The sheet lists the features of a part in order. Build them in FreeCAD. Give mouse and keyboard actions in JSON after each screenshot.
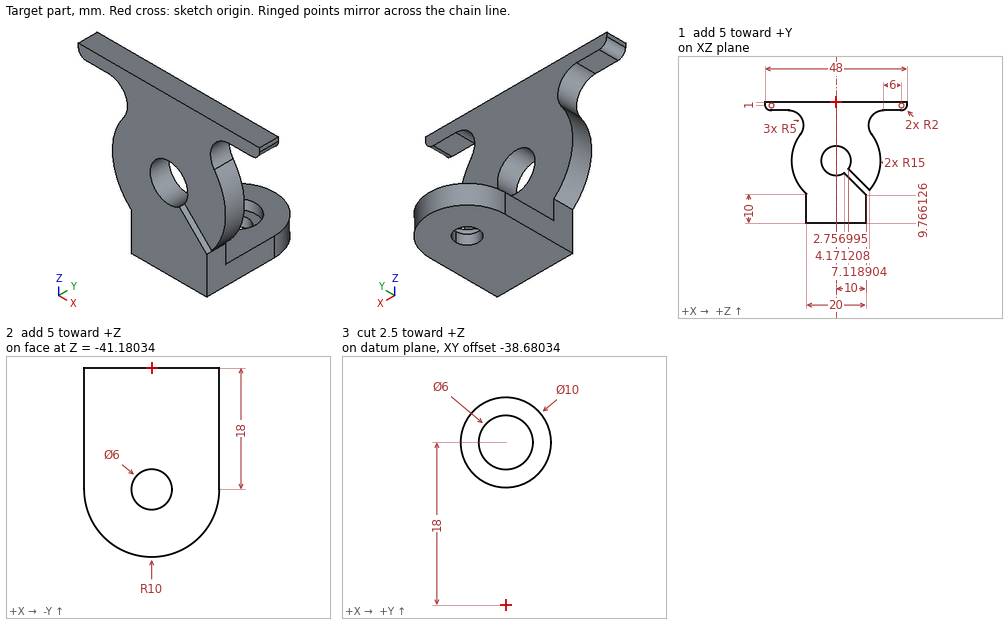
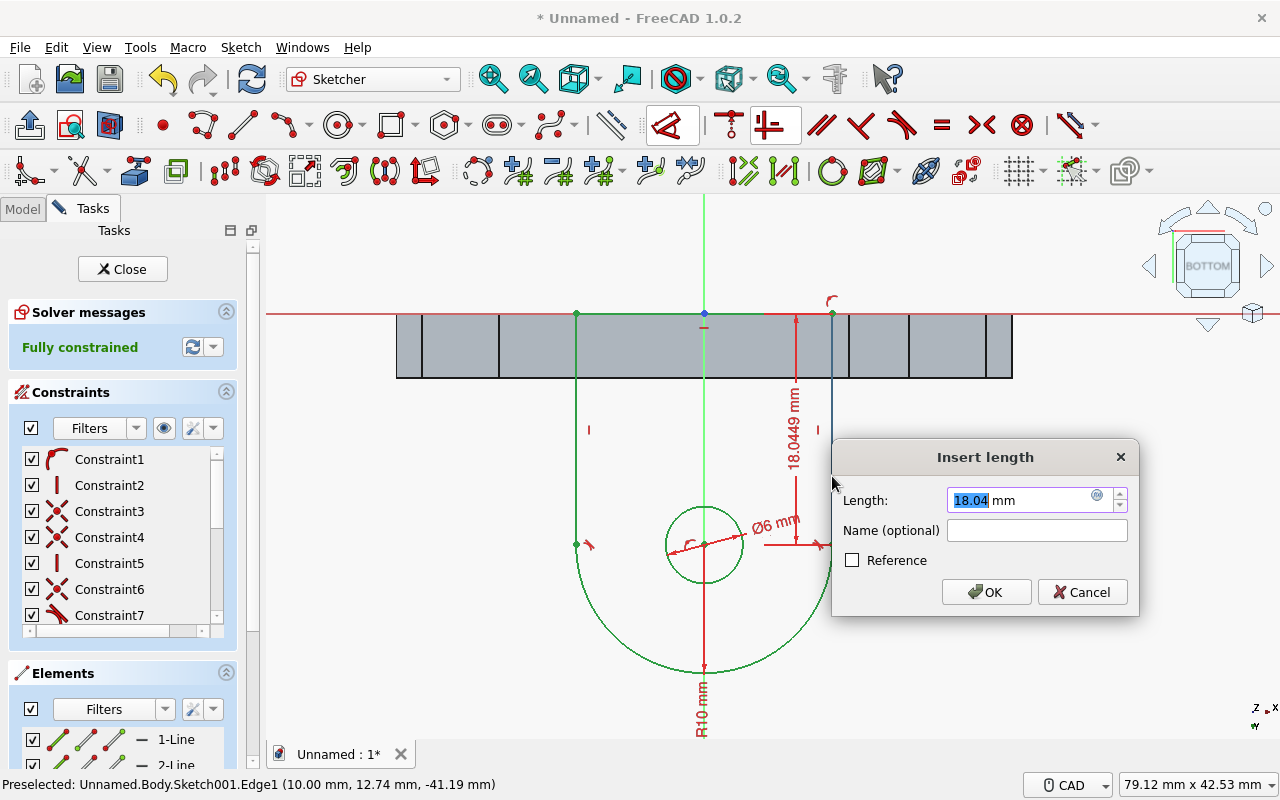
{"action": "type", "text": "18"}
{"action": "key", "text": "Return"}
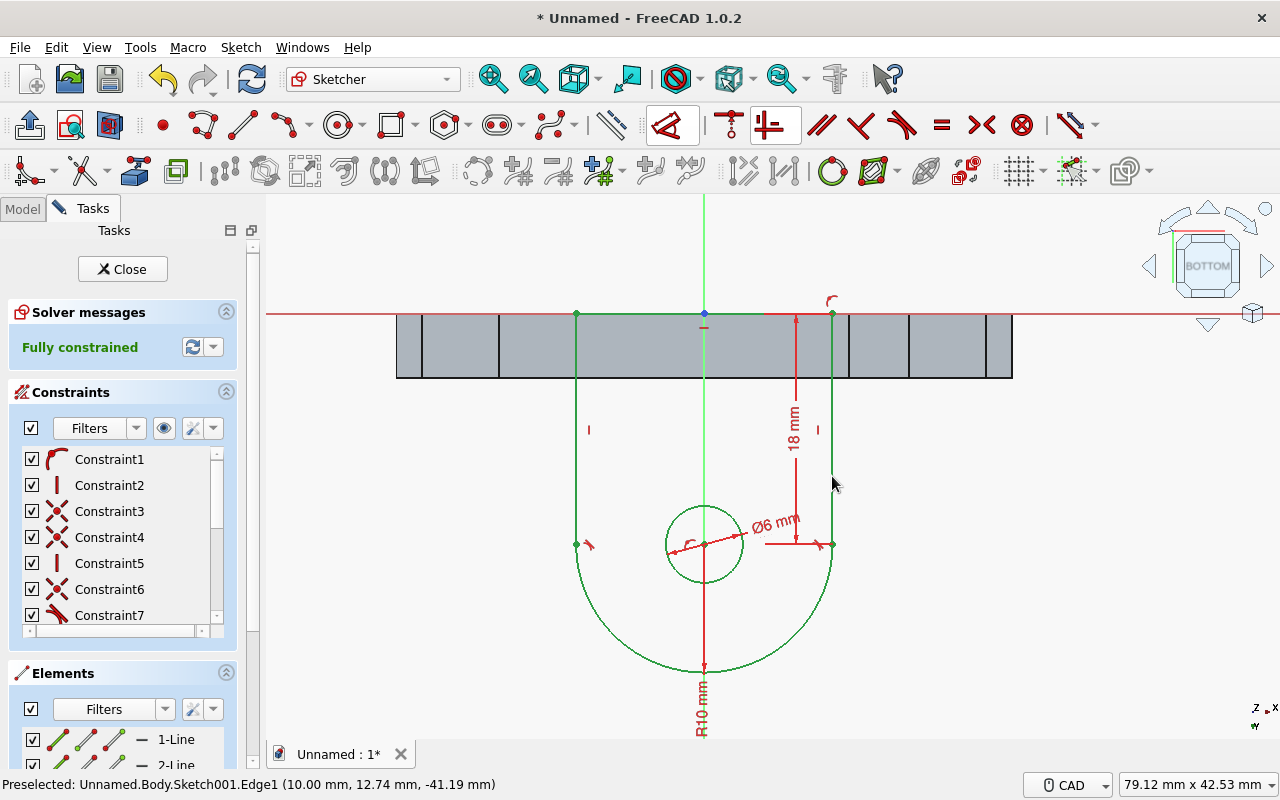
{"action": "left_click", "coordinate": [123, 269]}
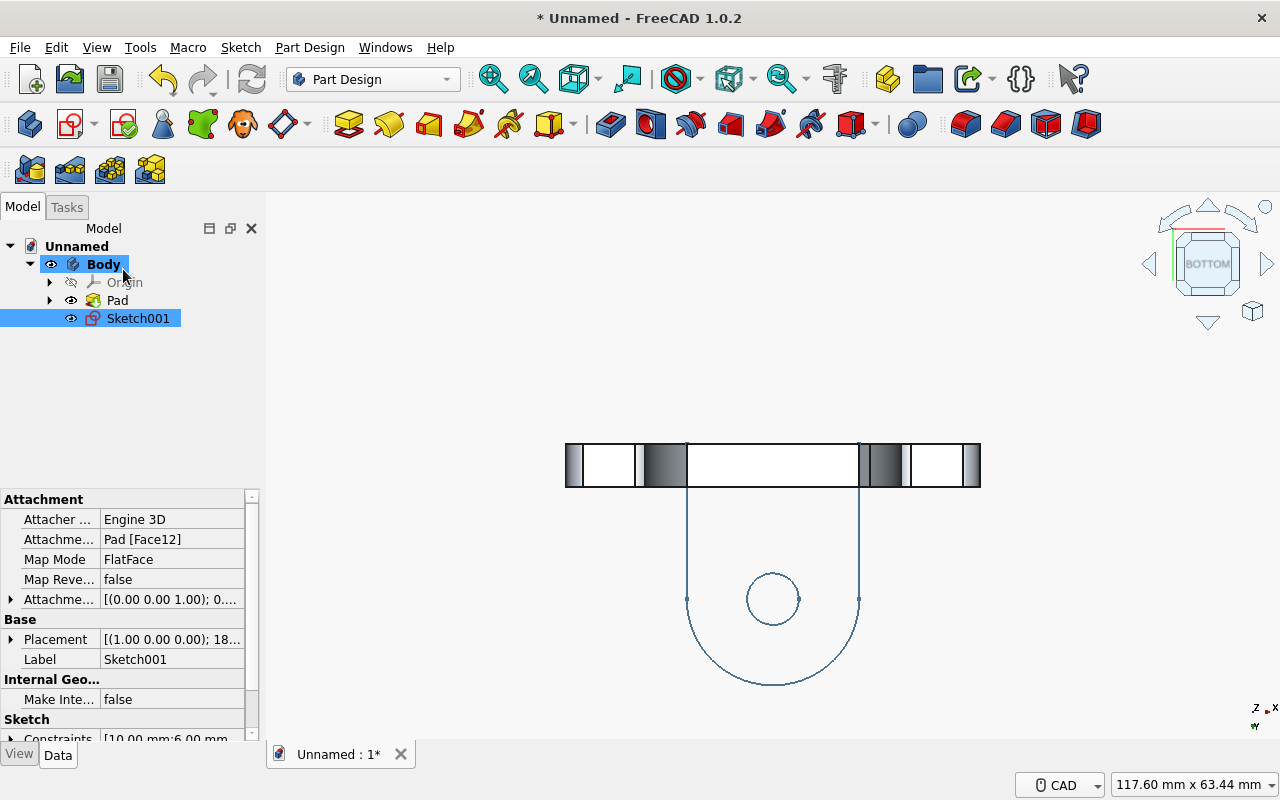
{"action": "left_click", "coordinate": [350, 124]}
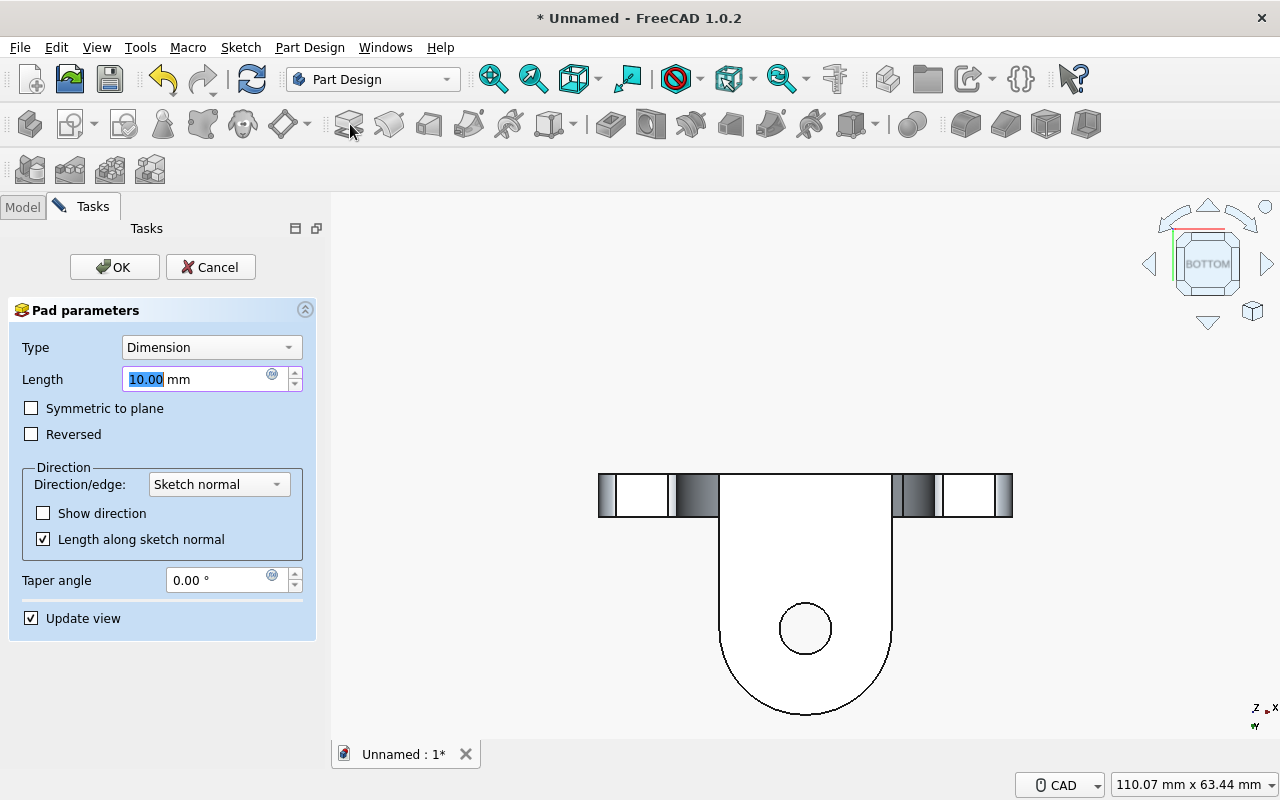
{"action": "type", "text": "5"}
{"action": "key", "text": "Tab"}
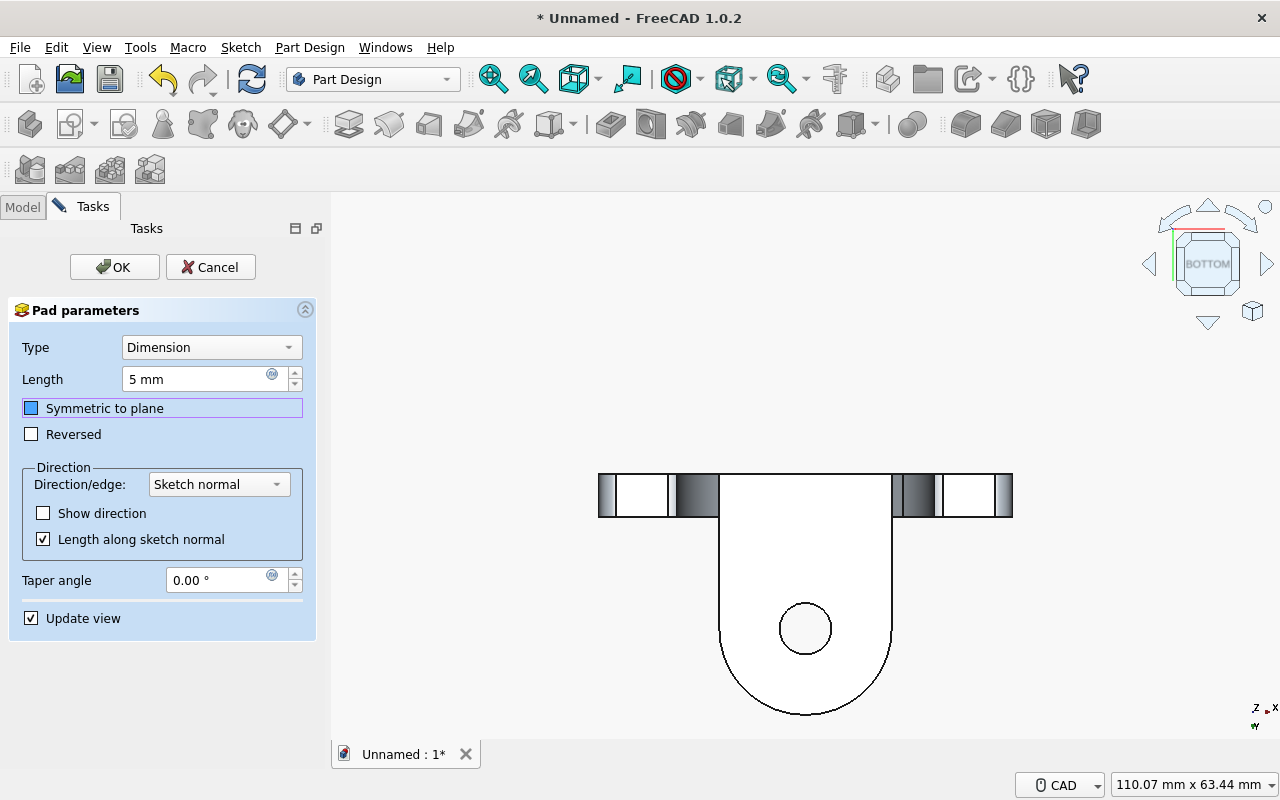
{"action": "left_click", "coordinate": [30, 434]}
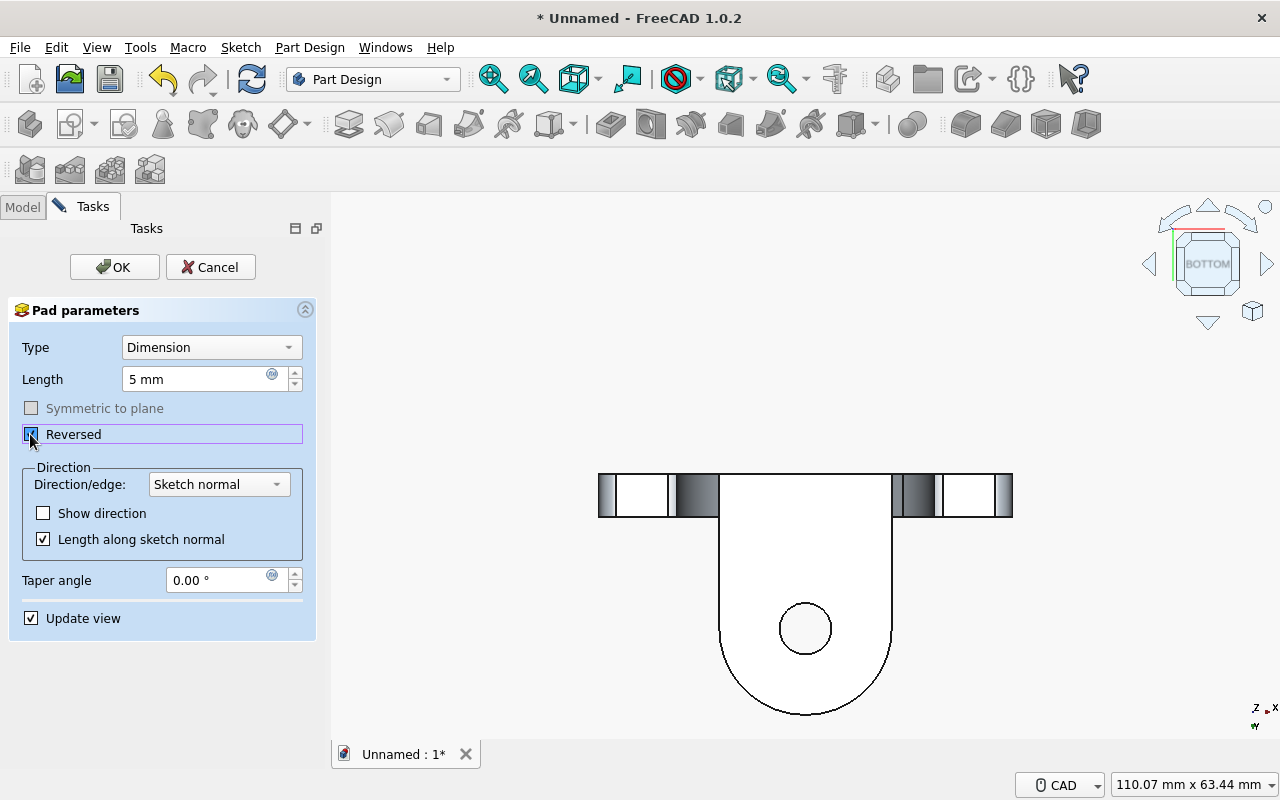
{"action": "left_click", "coordinate": [115, 267]}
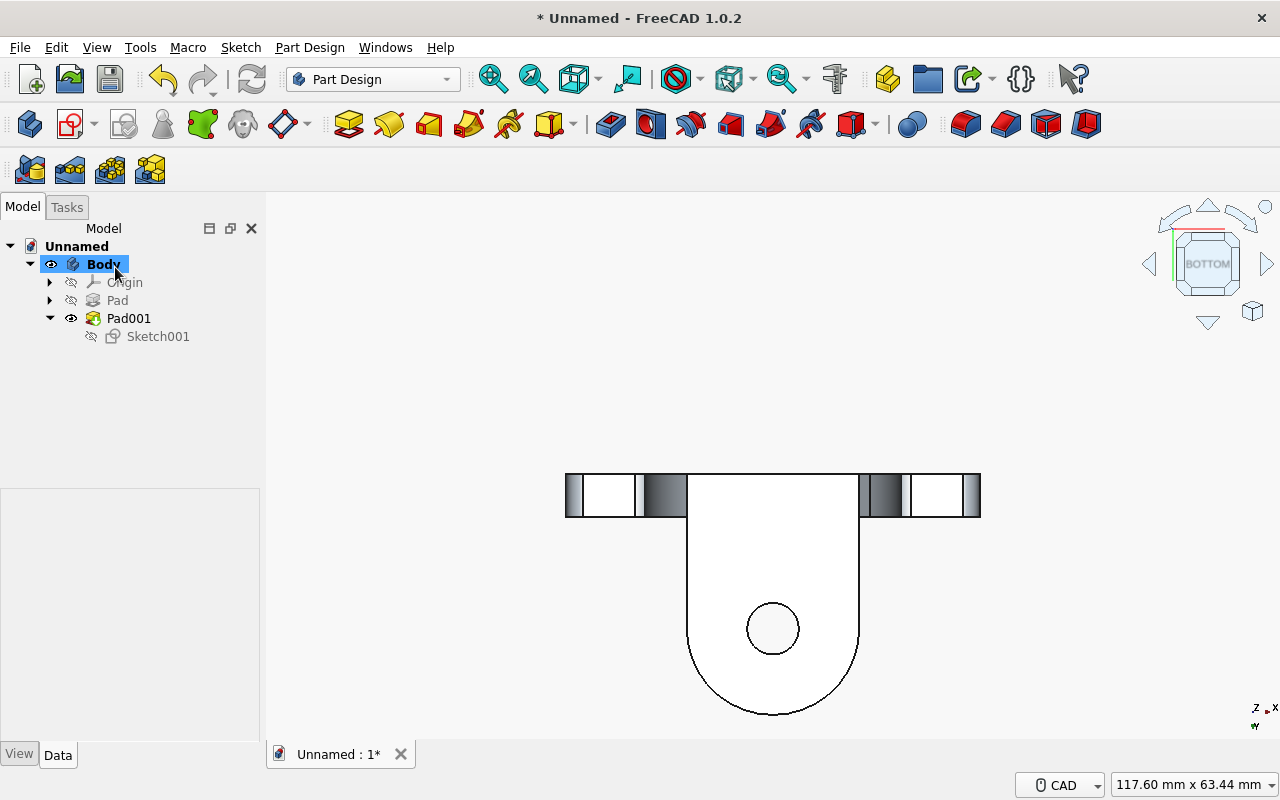
{"action": "left_click", "coordinate": [494, 80]}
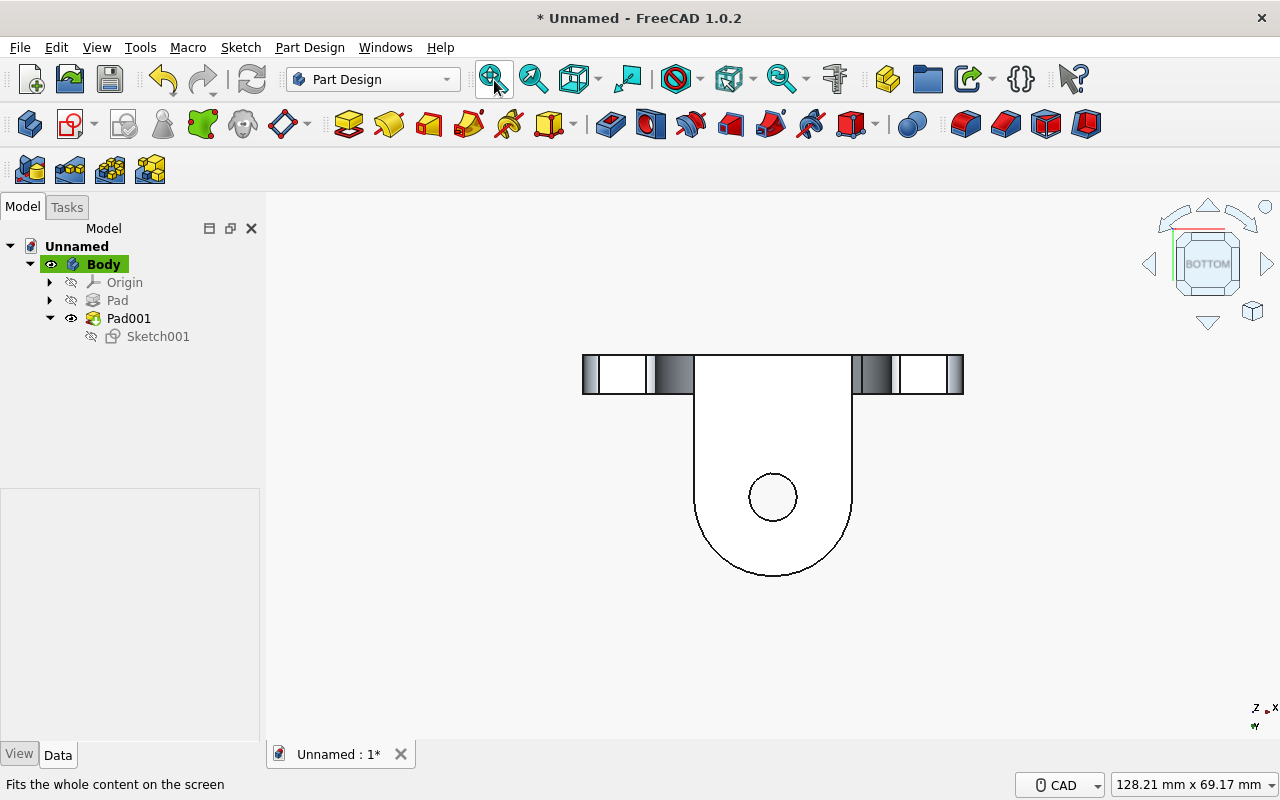
{"action": "left_click", "coordinate": [50, 282]}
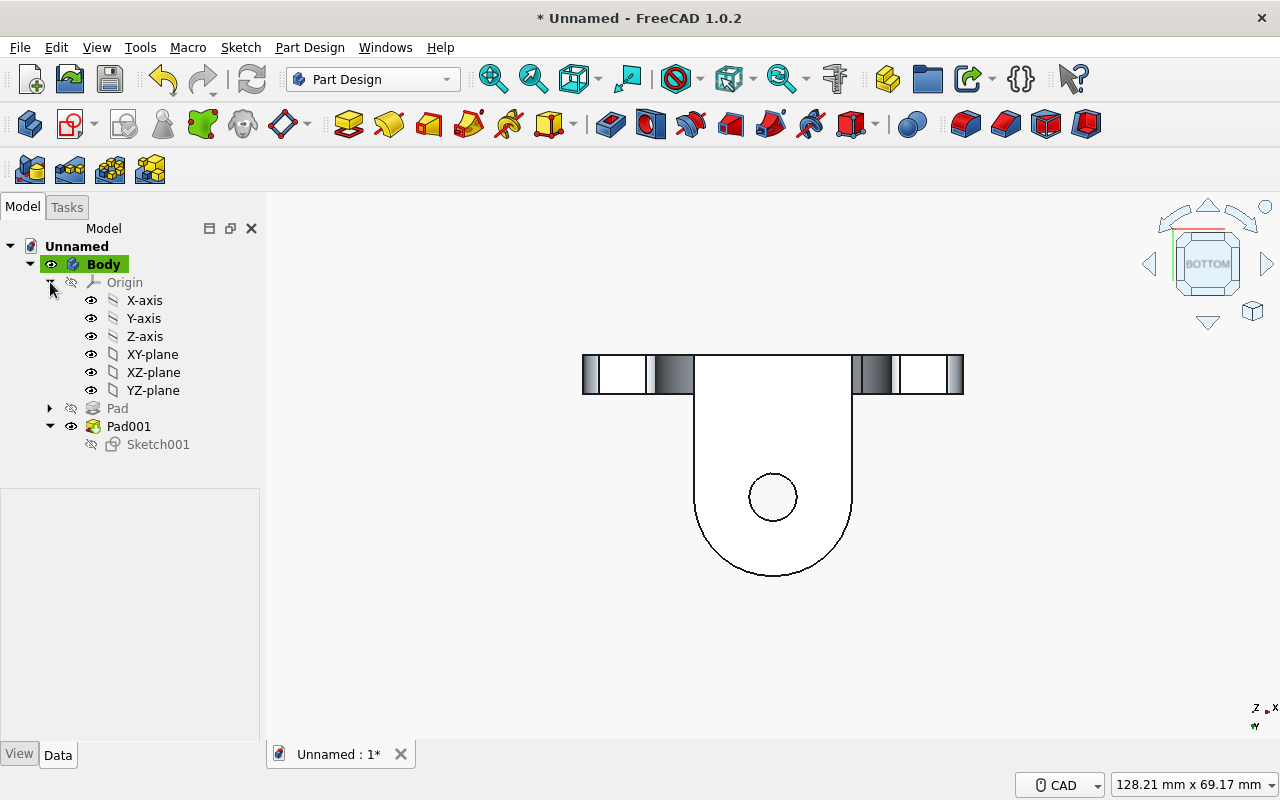
{"action": "left_click", "coordinate": [136, 354]}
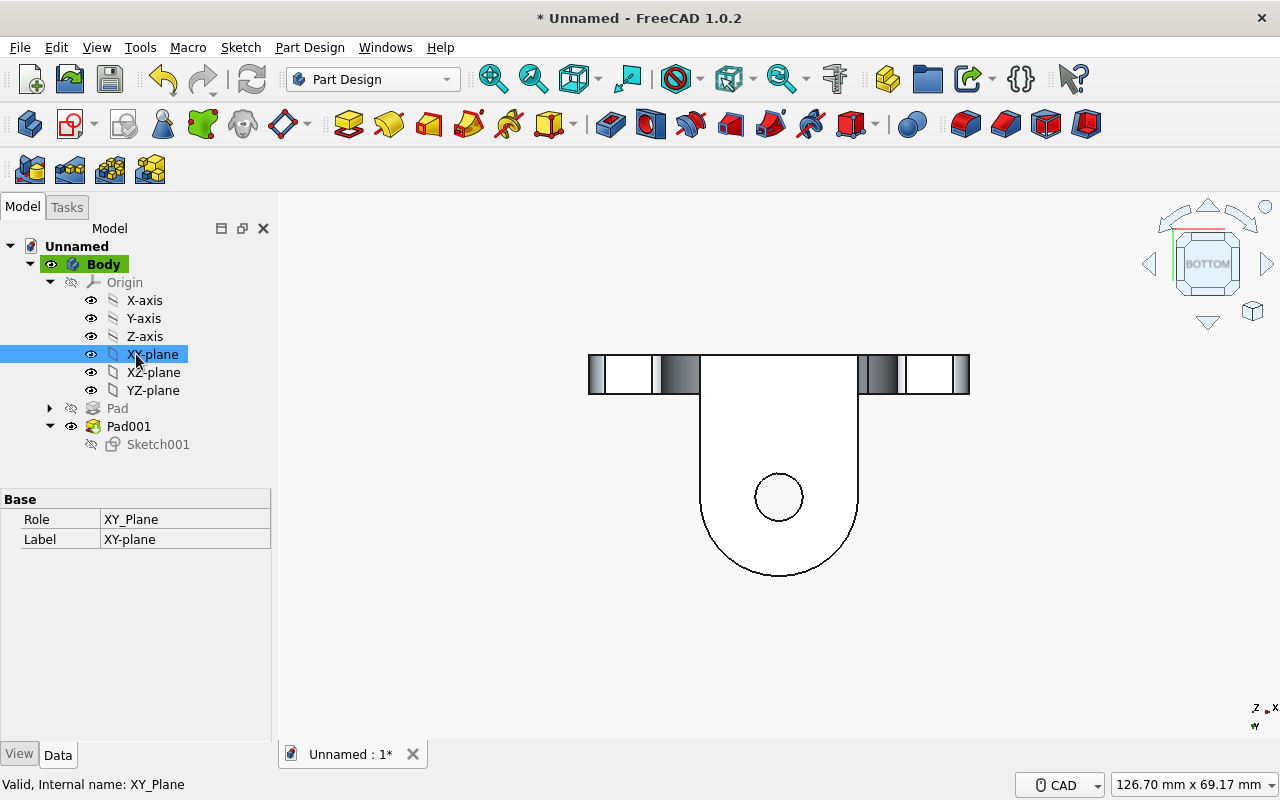
{"action": "left_click", "coordinate": [284, 124]}